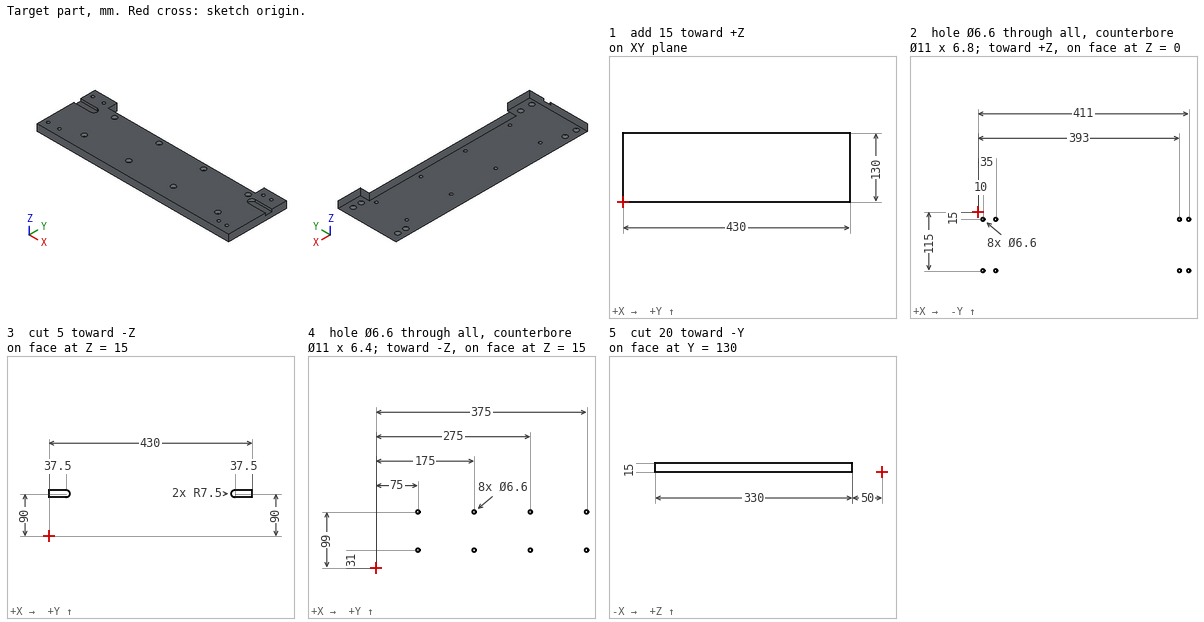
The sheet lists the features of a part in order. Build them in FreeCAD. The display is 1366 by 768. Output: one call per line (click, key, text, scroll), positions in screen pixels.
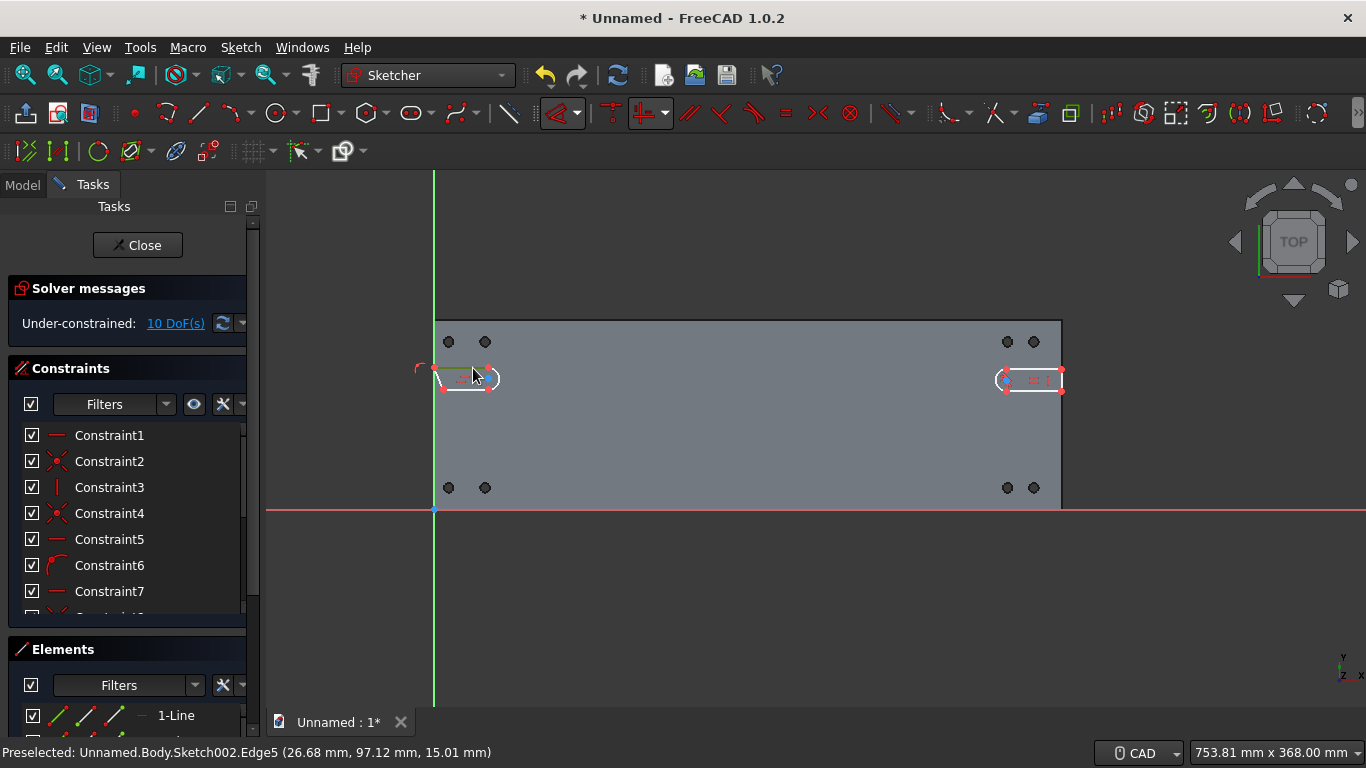
scroll(497, 385, up, 2)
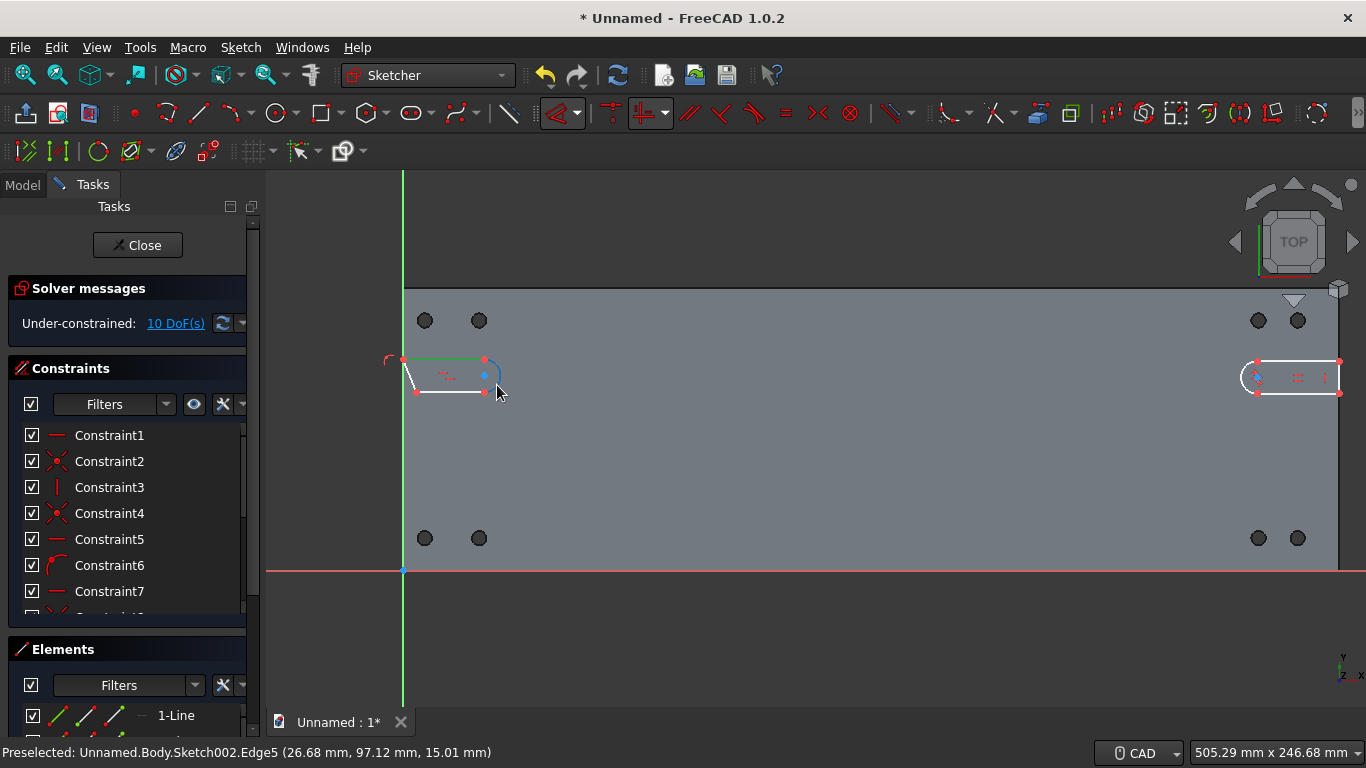
click(498, 385)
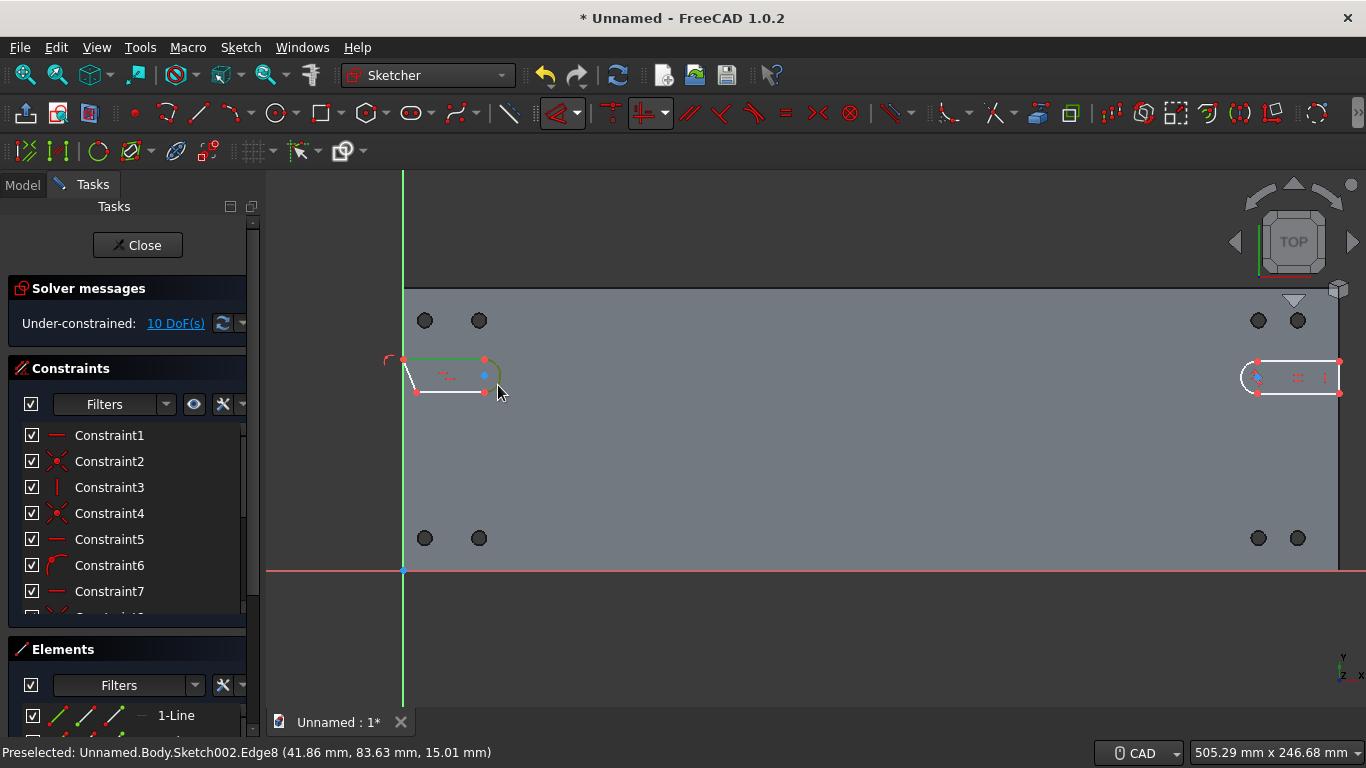
click(754, 114)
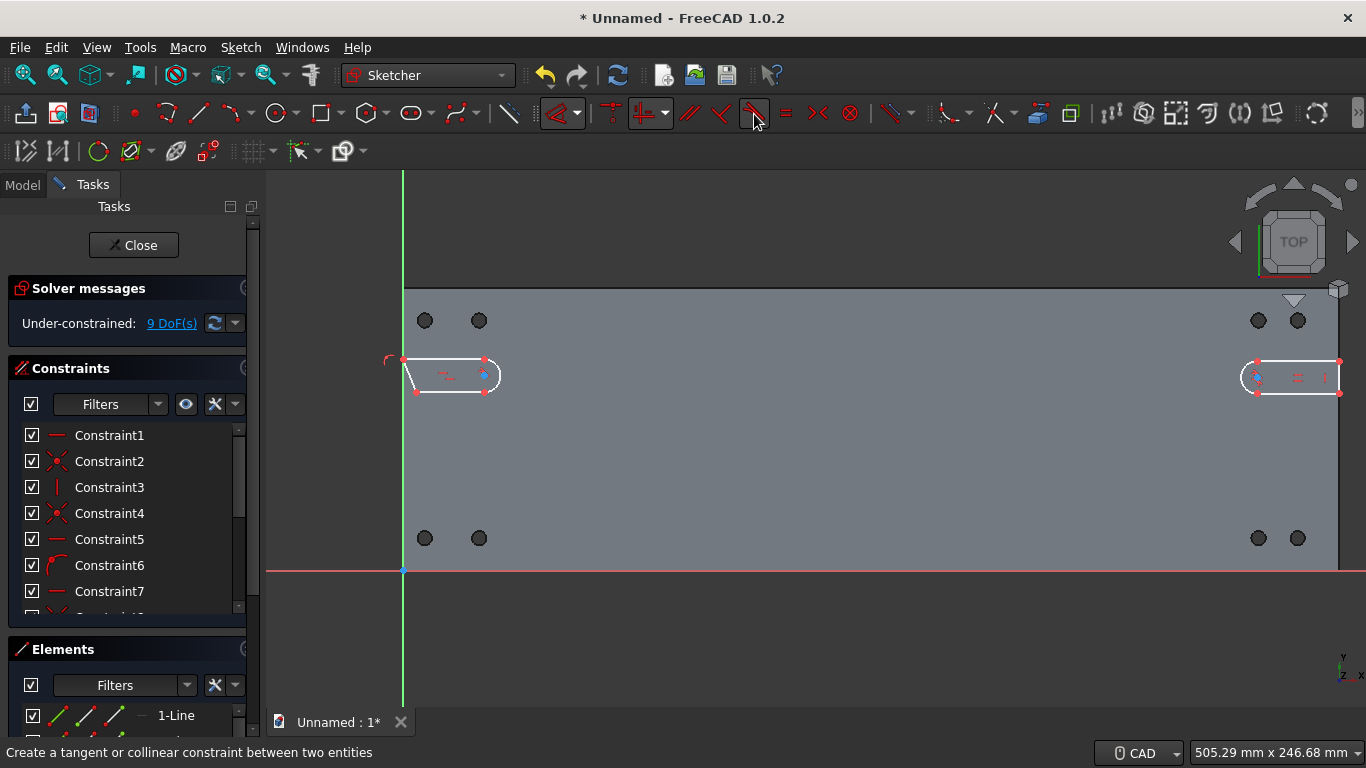
click(437, 392)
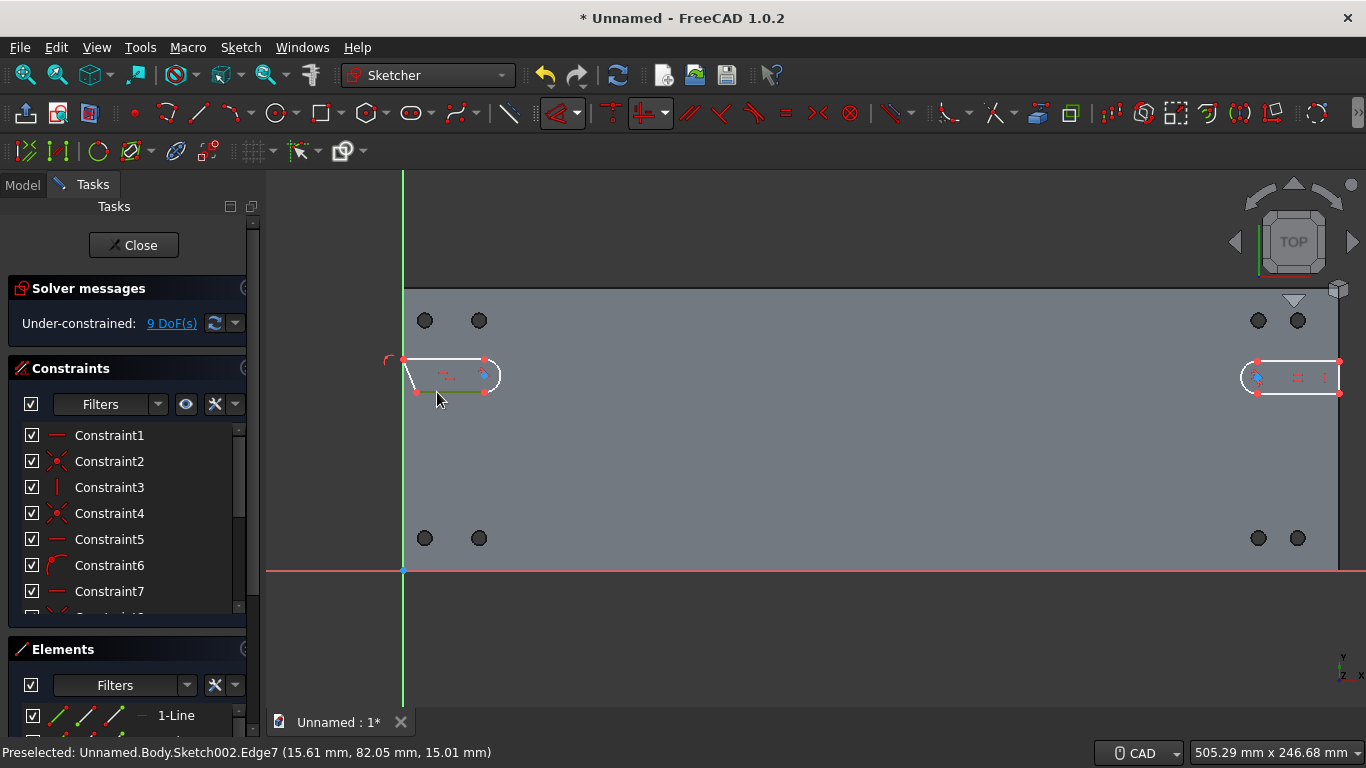
click(498, 385)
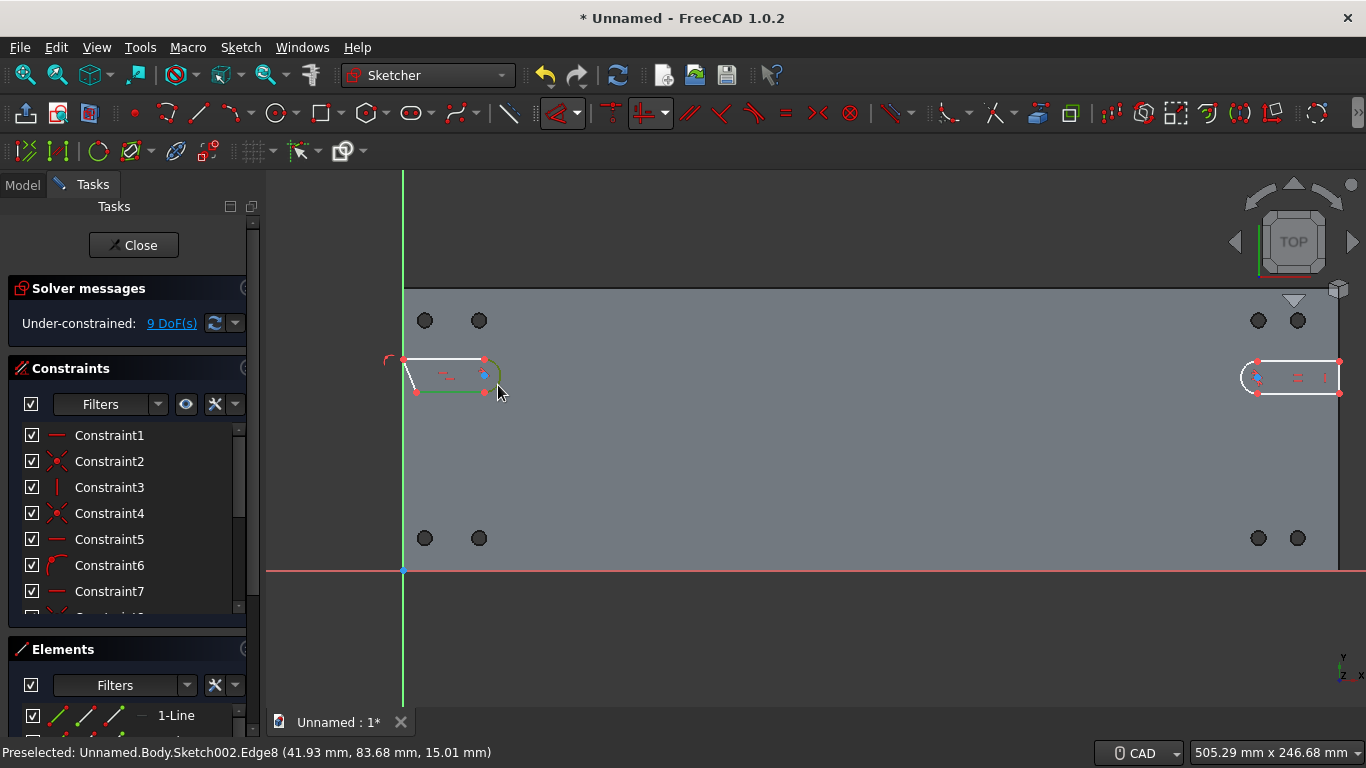
click(754, 114)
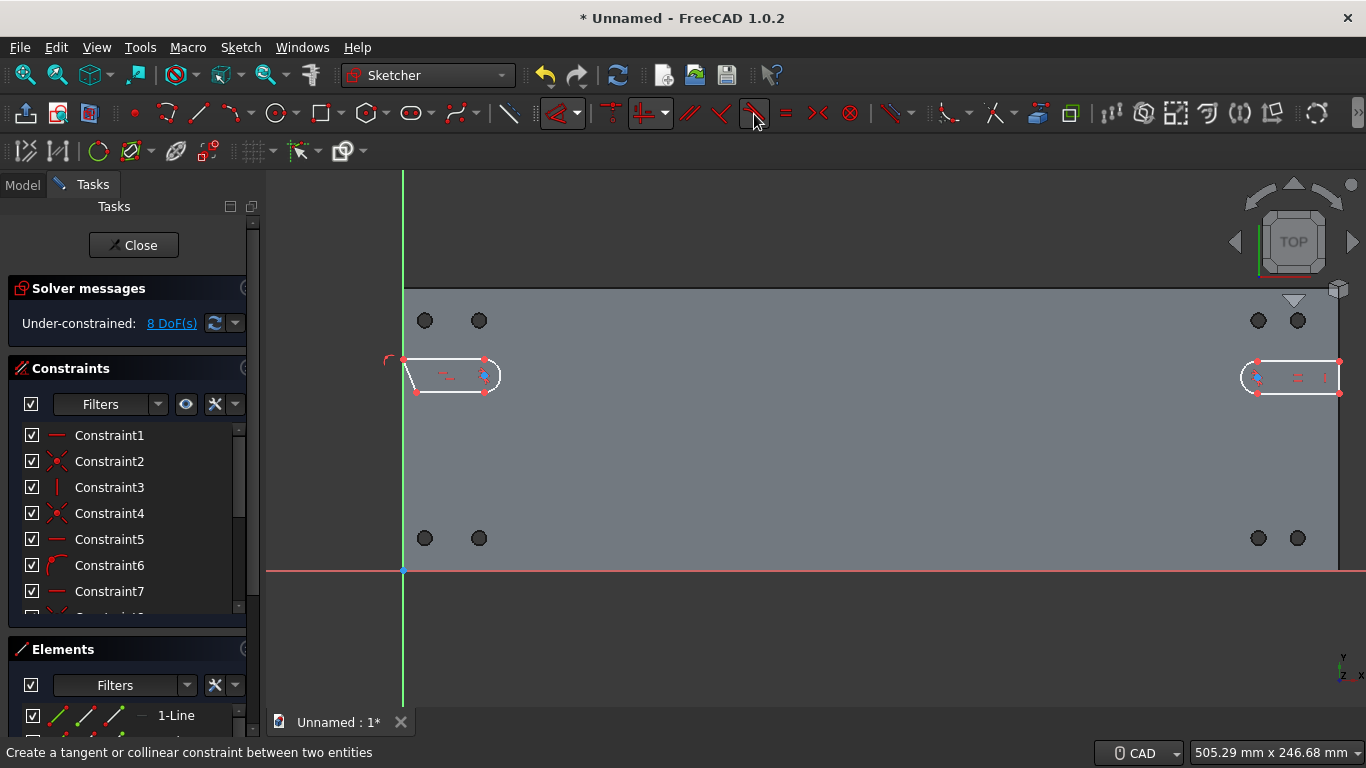
scroll(407, 369, up, 2)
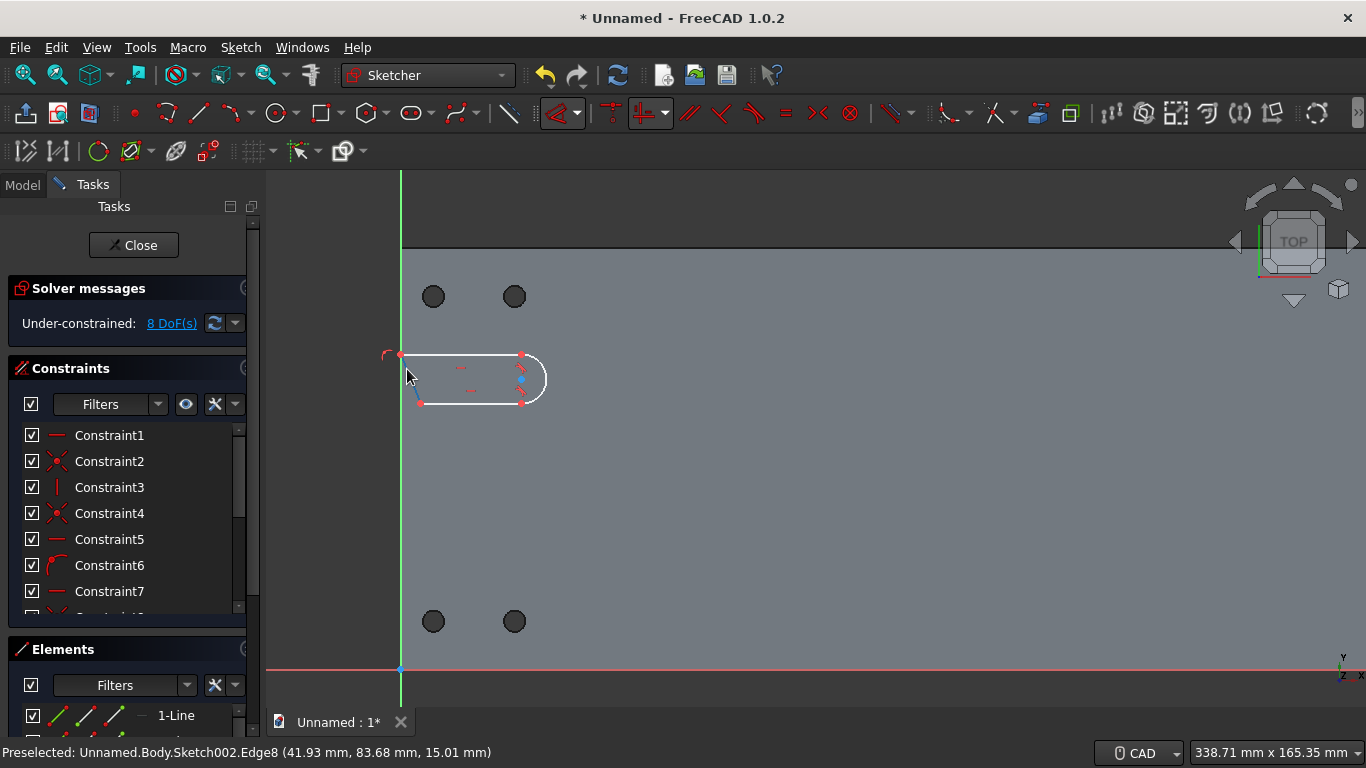
click(407, 369)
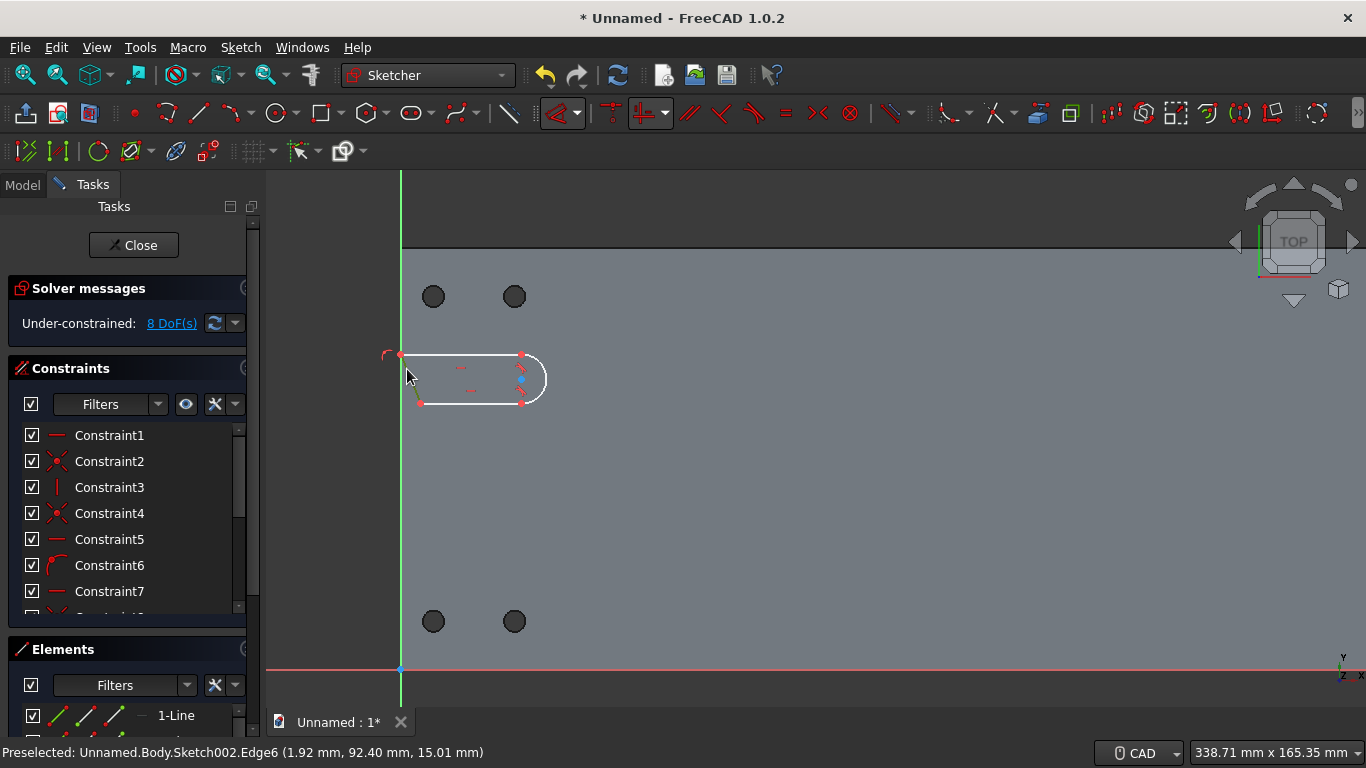
click(668, 114)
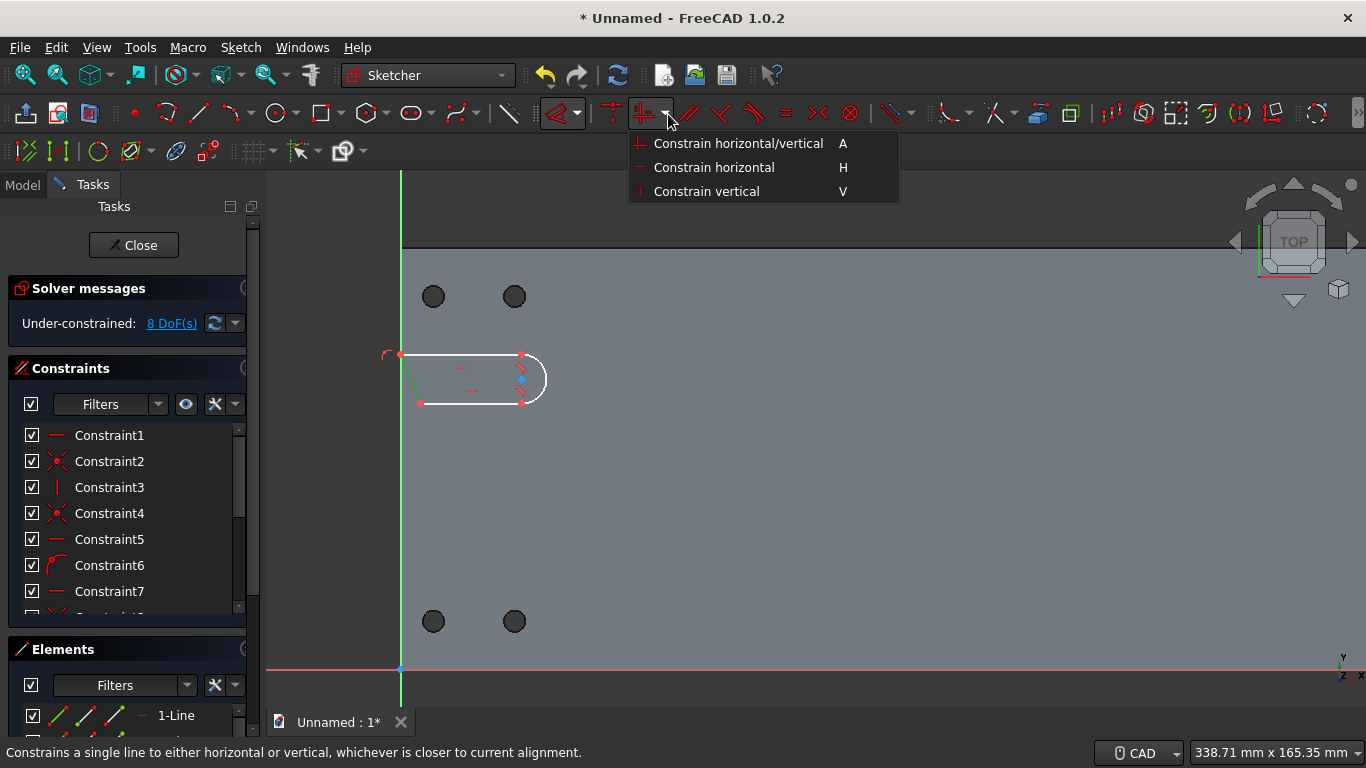
click(764, 191)